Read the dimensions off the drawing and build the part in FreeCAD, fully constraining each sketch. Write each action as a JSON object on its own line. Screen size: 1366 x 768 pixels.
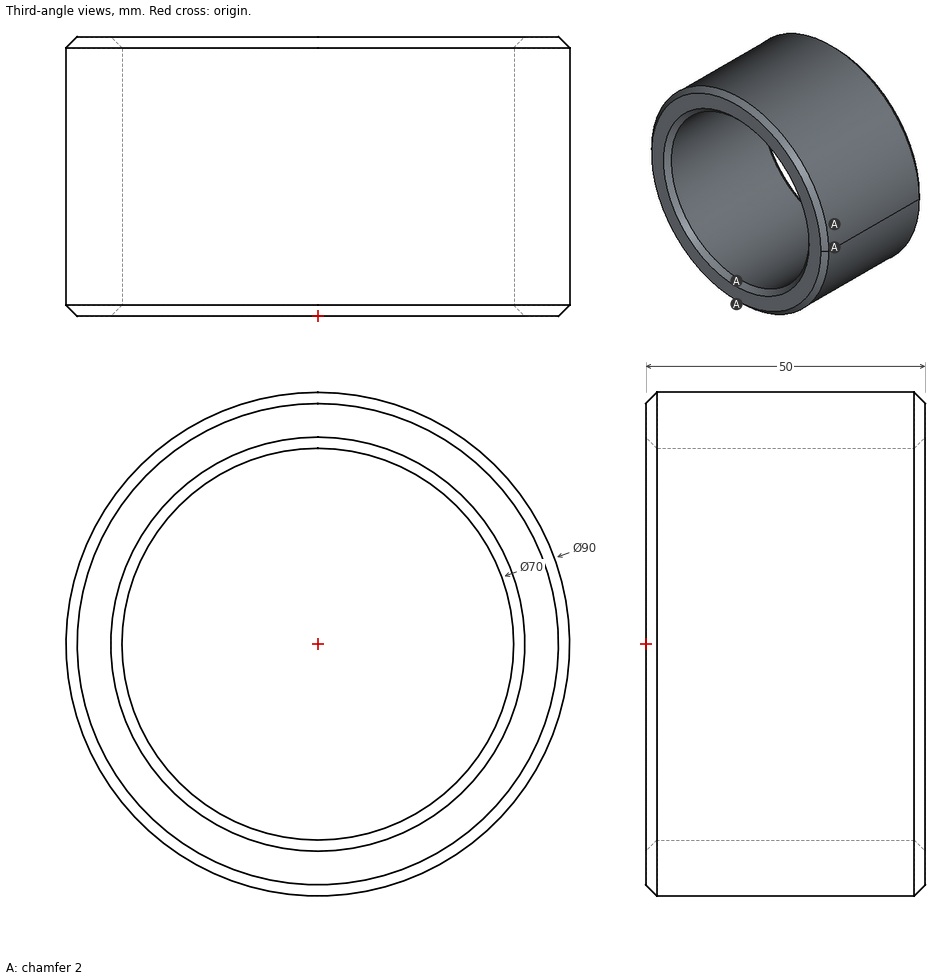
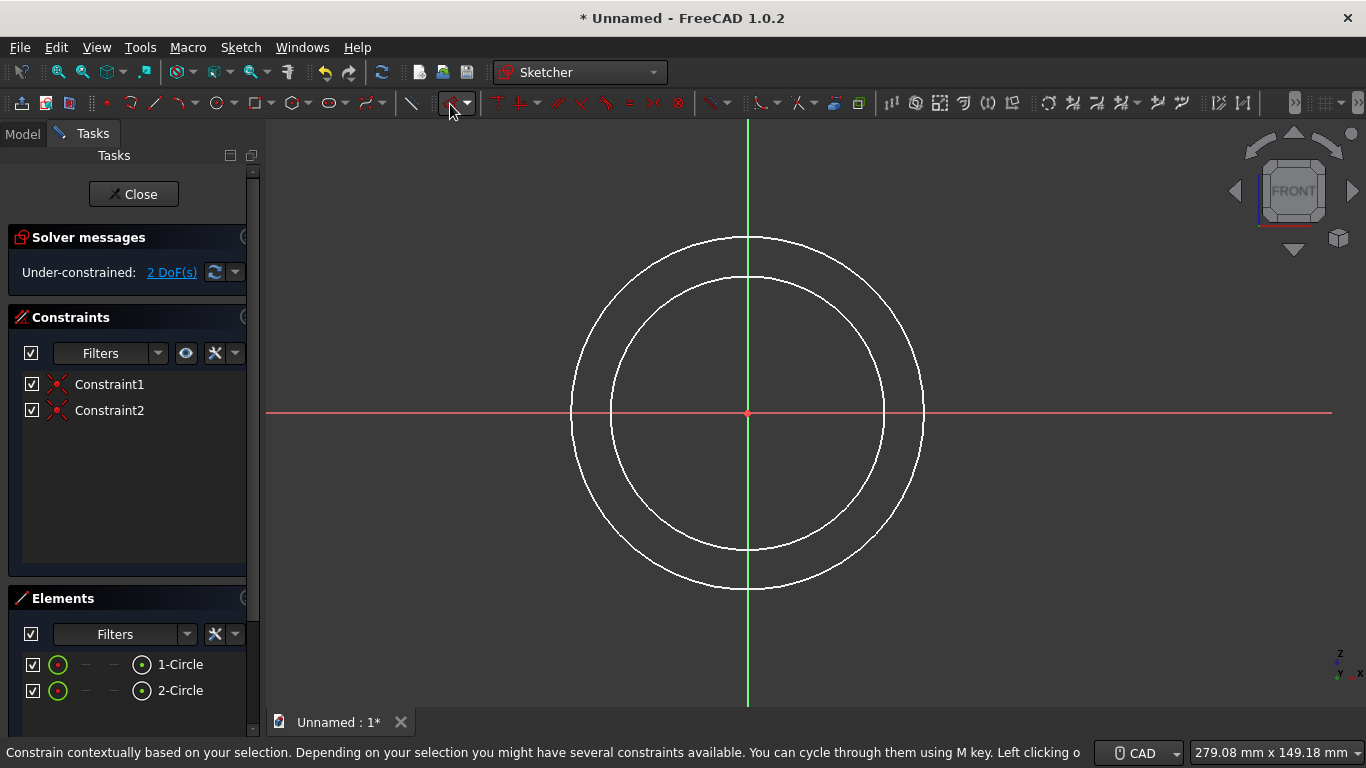
{"action": "left_click", "coordinate": [872, 288]}
{"action": "left_click", "coordinate": [895, 265]}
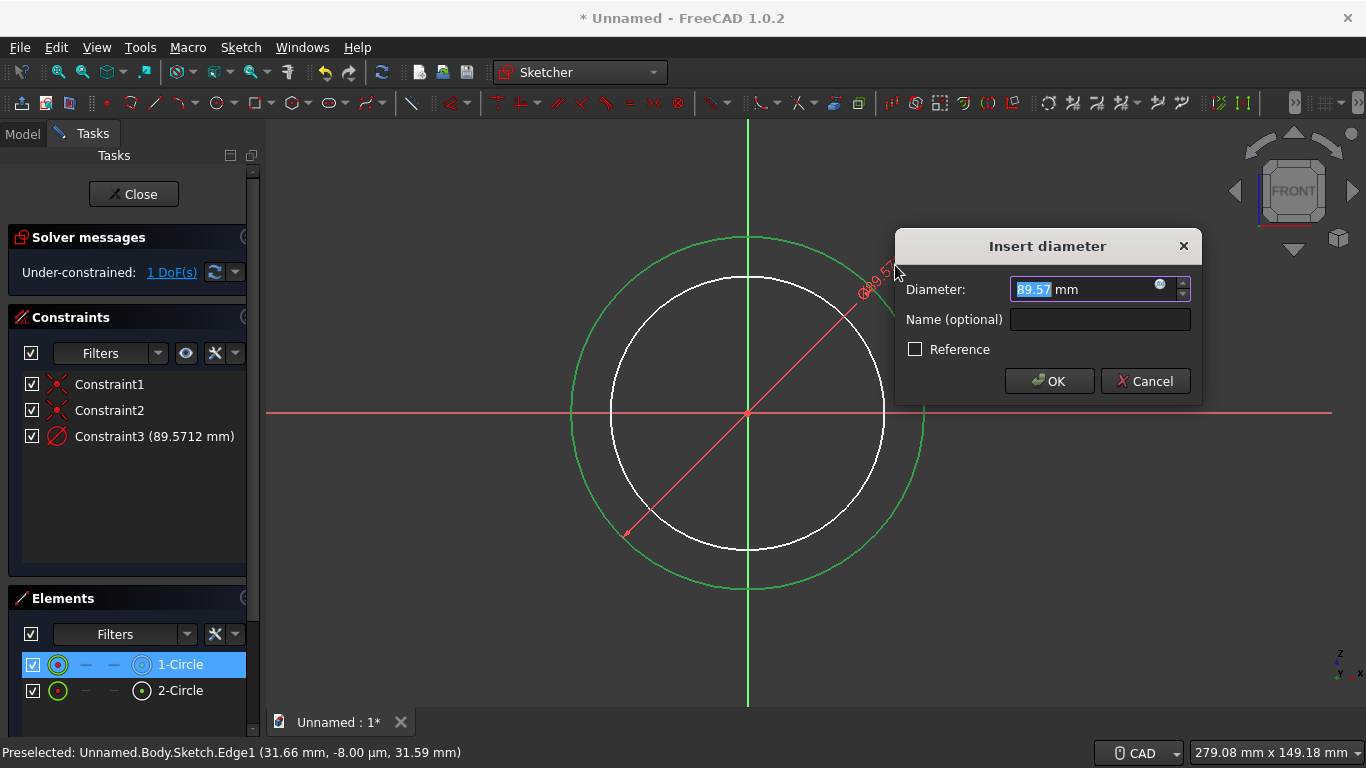
{"action": "type", "text": "90"}
{"action": "key", "text": "Return"}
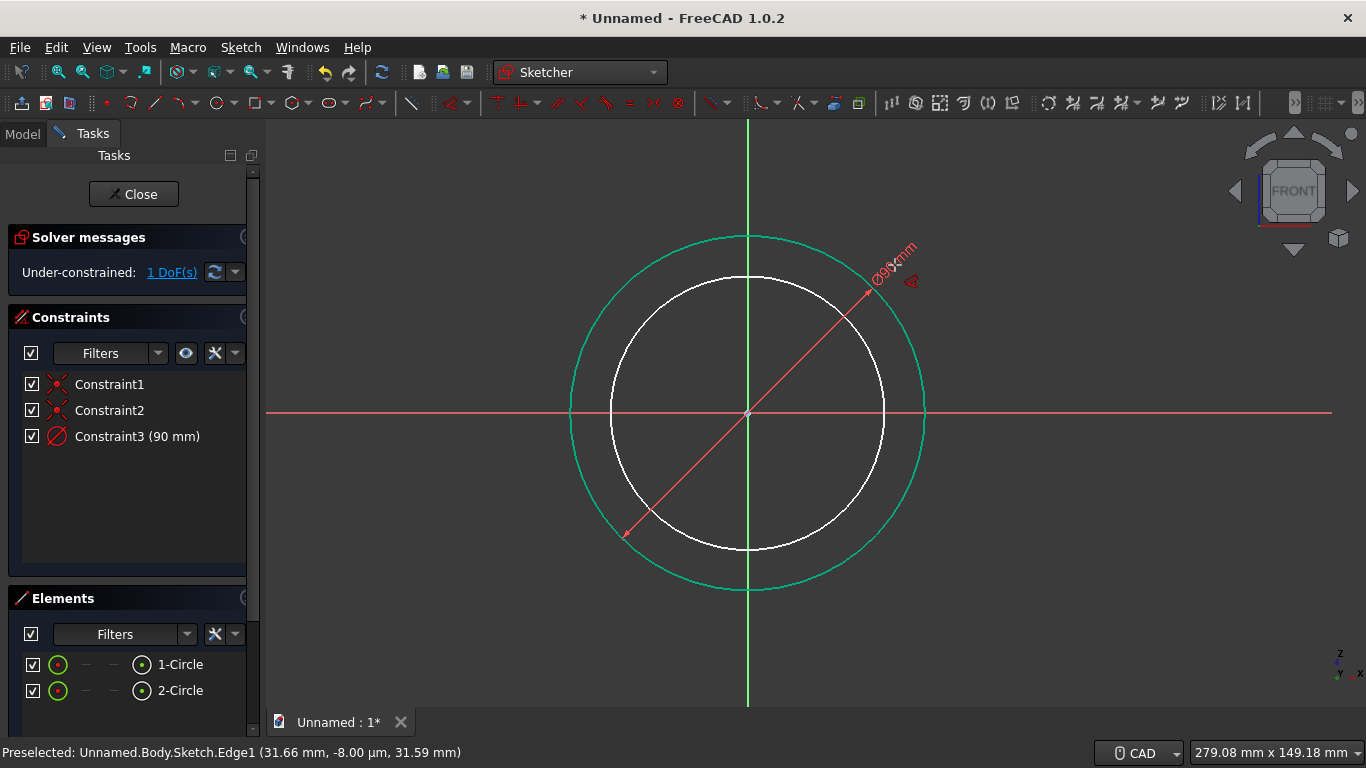
{"action": "left_click", "coordinate": [844, 316]}
{"action": "left_click", "coordinate": [931, 358]}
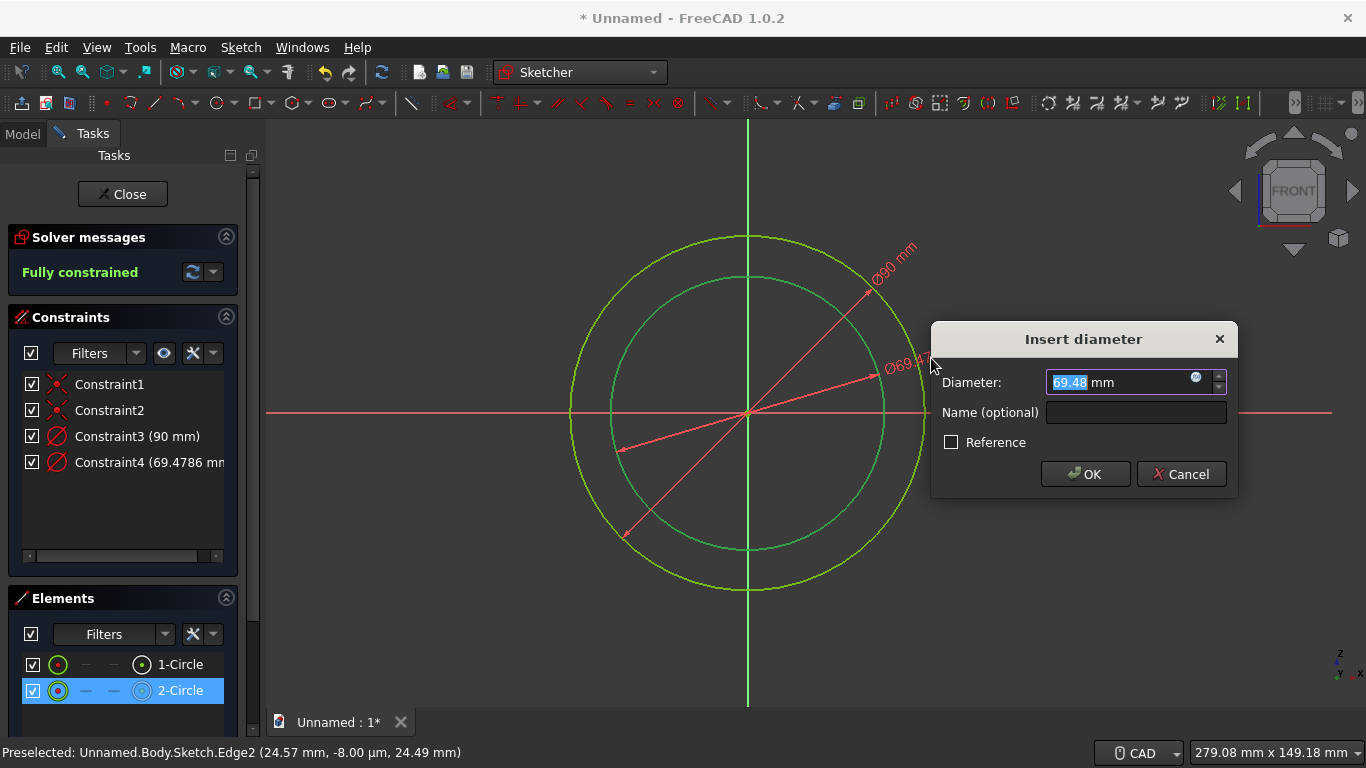
{"action": "type", "text": "70"}
{"action": "key", "text": "Return"}
{"action": "key", "text": "Escape"}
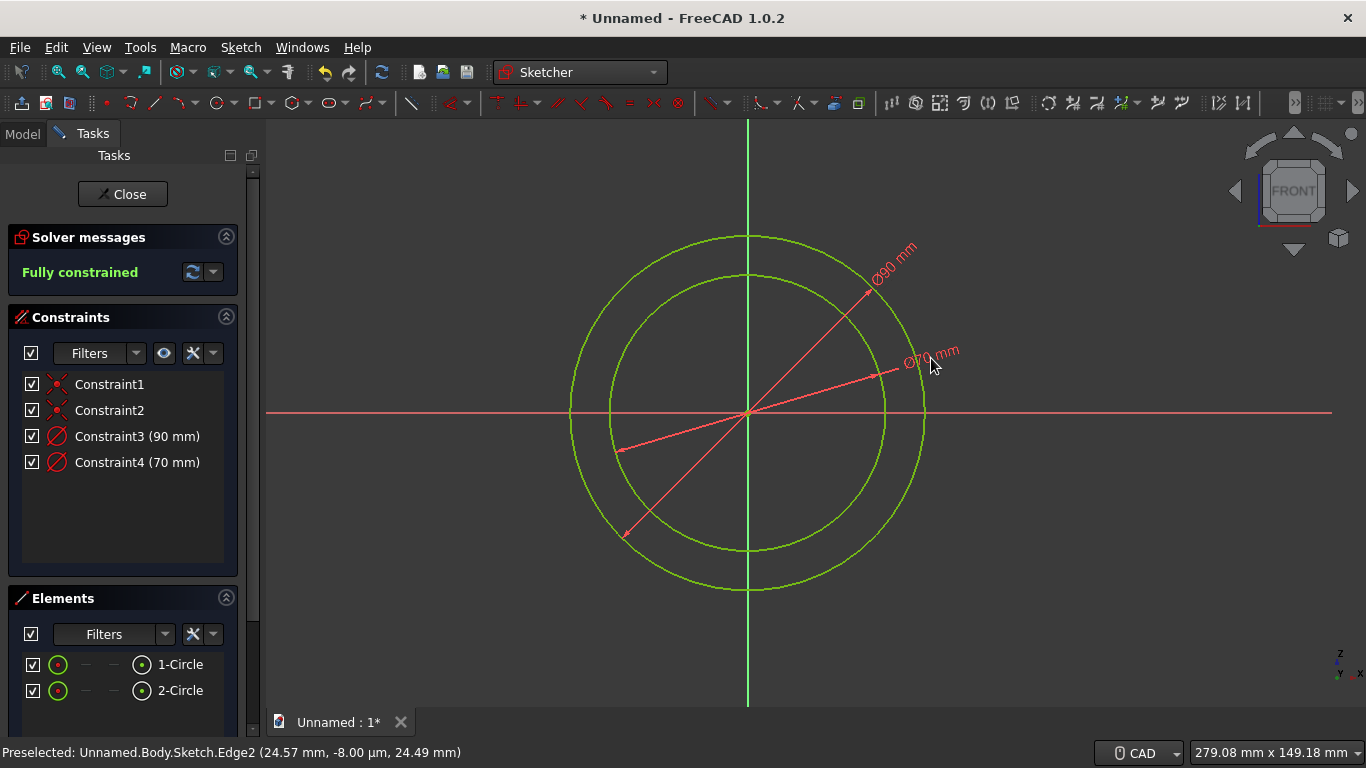
{"action": "left_click", "coordinate": [123, 194]}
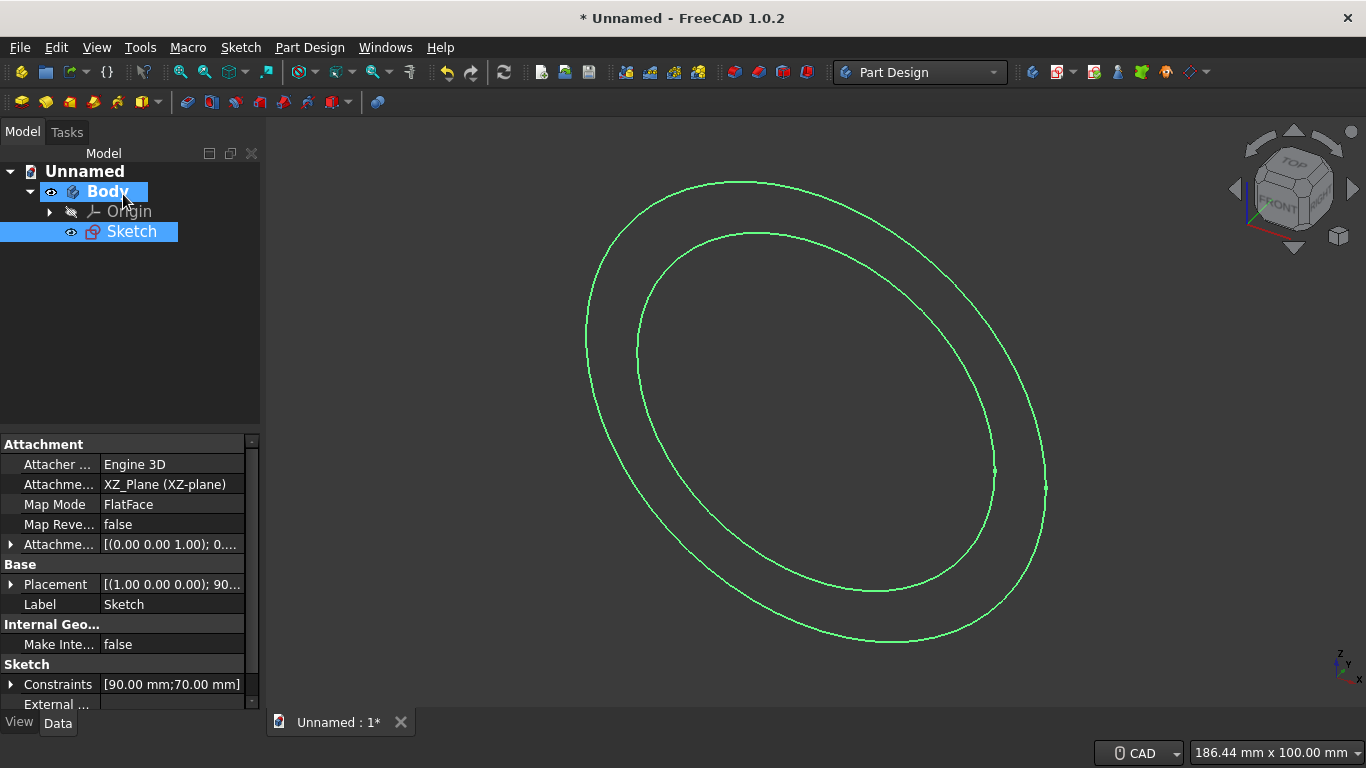
{"action": "left_click", "coordinate": [22, 102]}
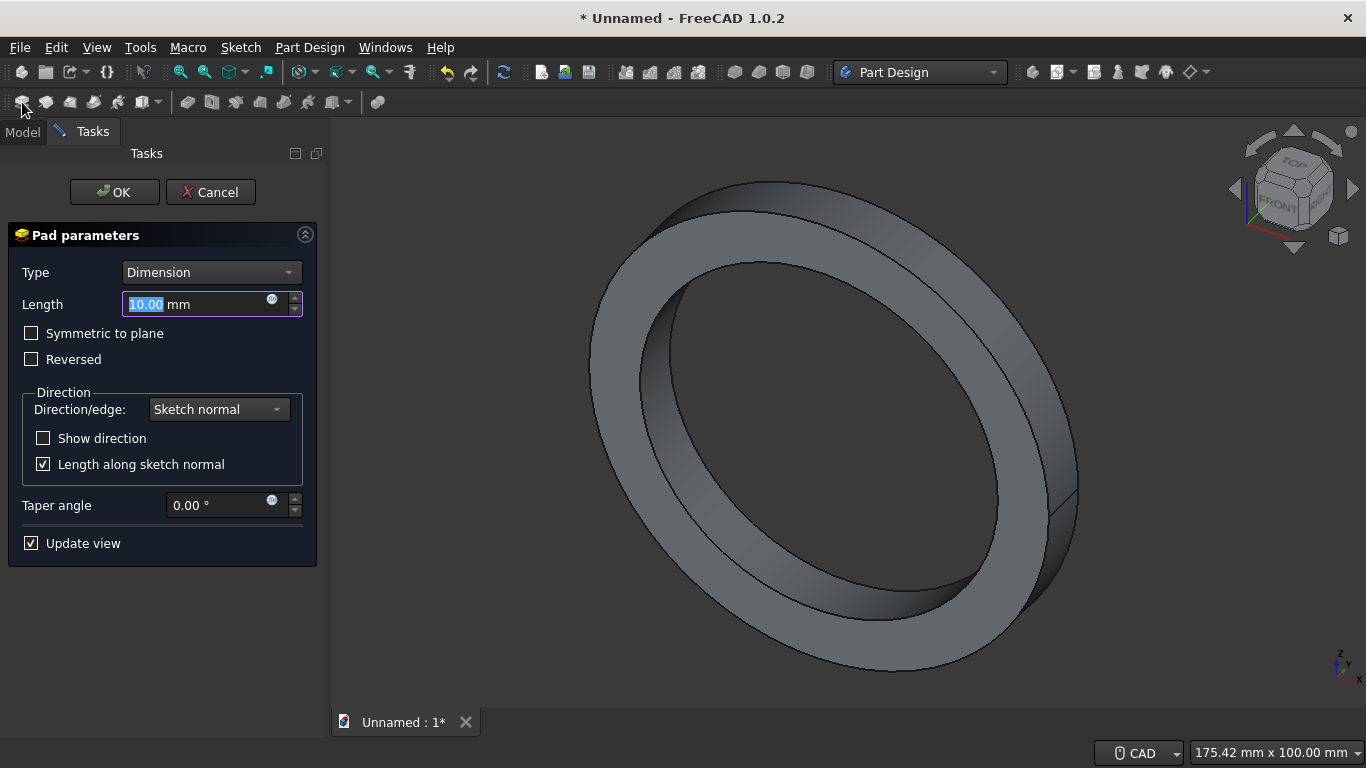
{"action": "type", "text": "50"}
{"action": "key", "text": "Tab"}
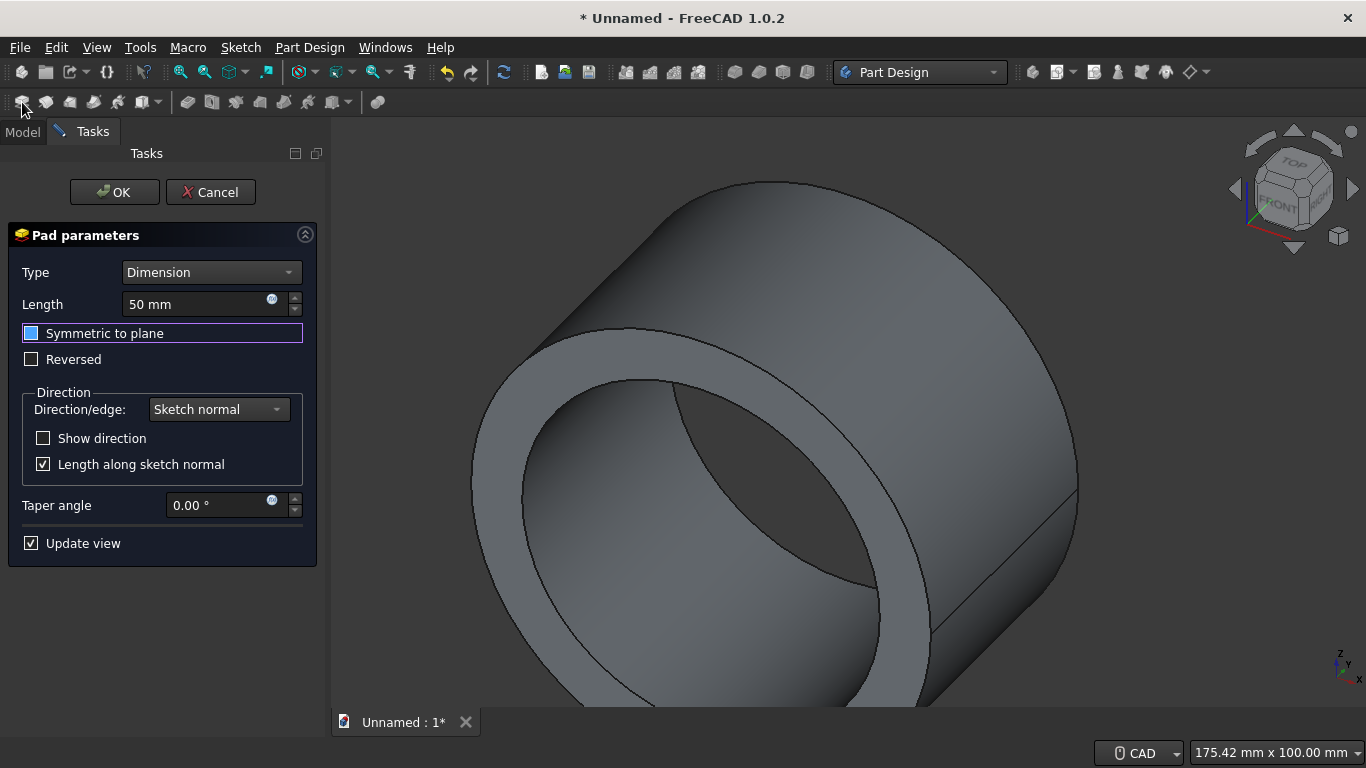
{"action": "left_click", "coordinate": [30, 359]}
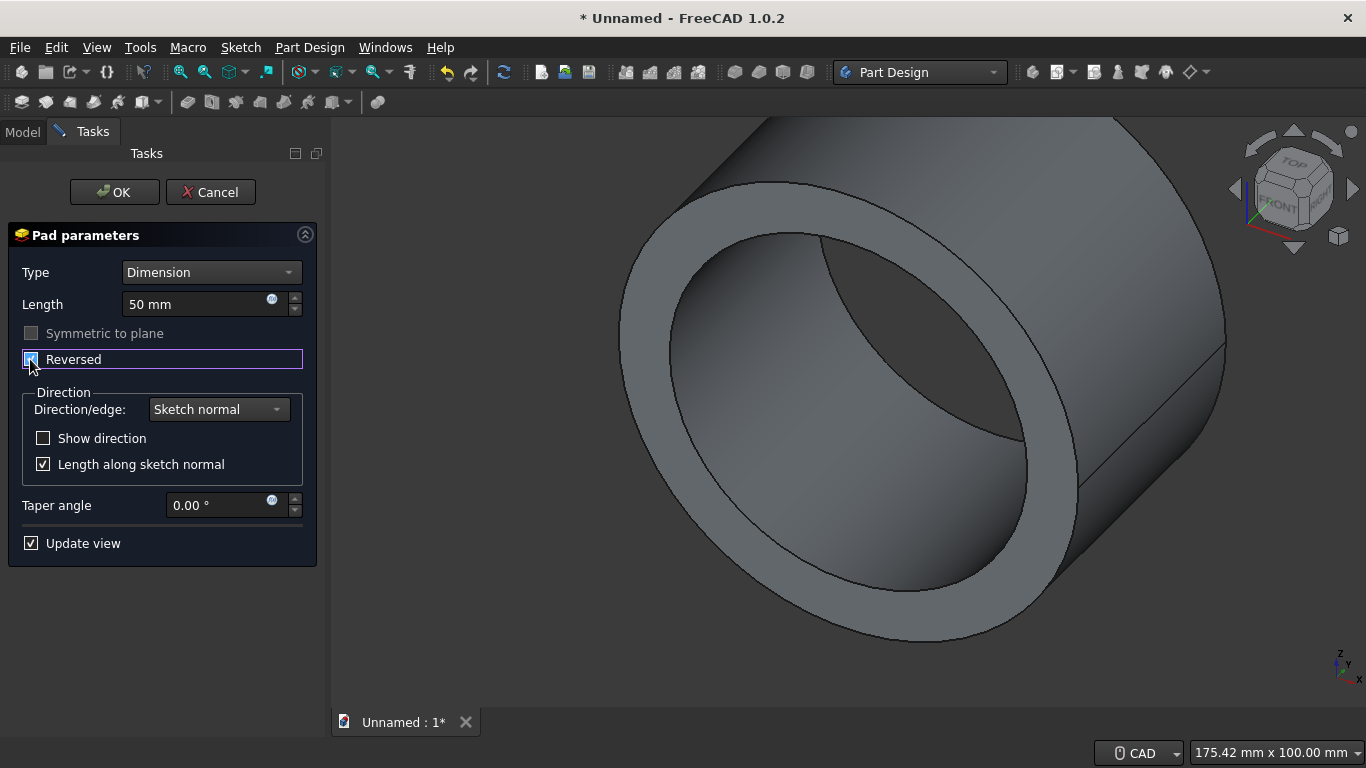
{"action": "left_click", "coordinate": [115, 192]}